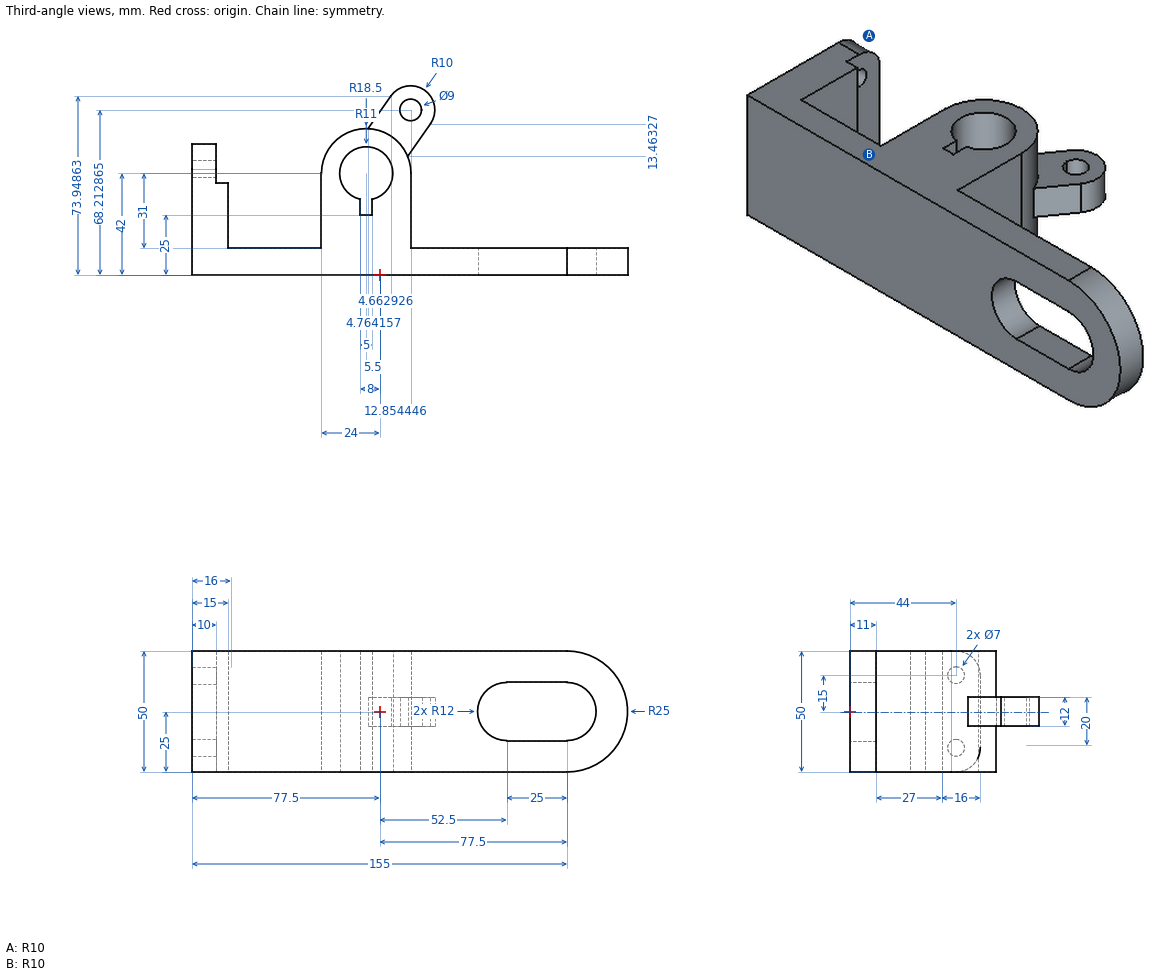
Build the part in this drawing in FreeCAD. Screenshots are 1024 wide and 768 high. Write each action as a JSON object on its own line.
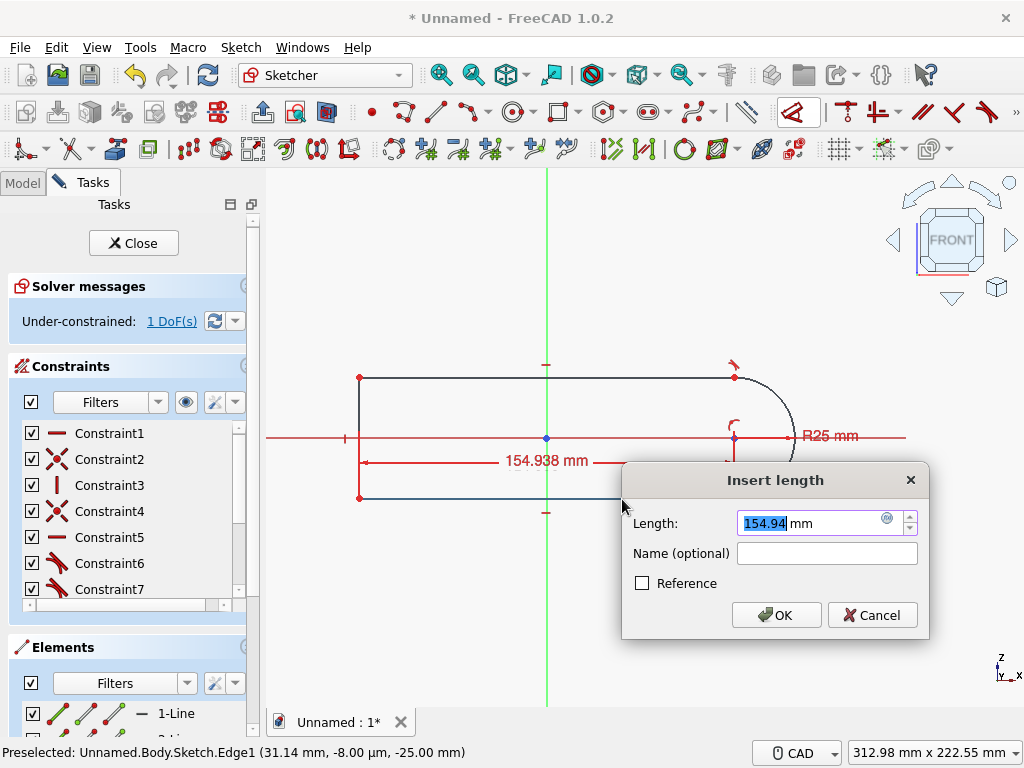
{"action": "type", "text": "155"}
{"action": "key", "text": "Return"}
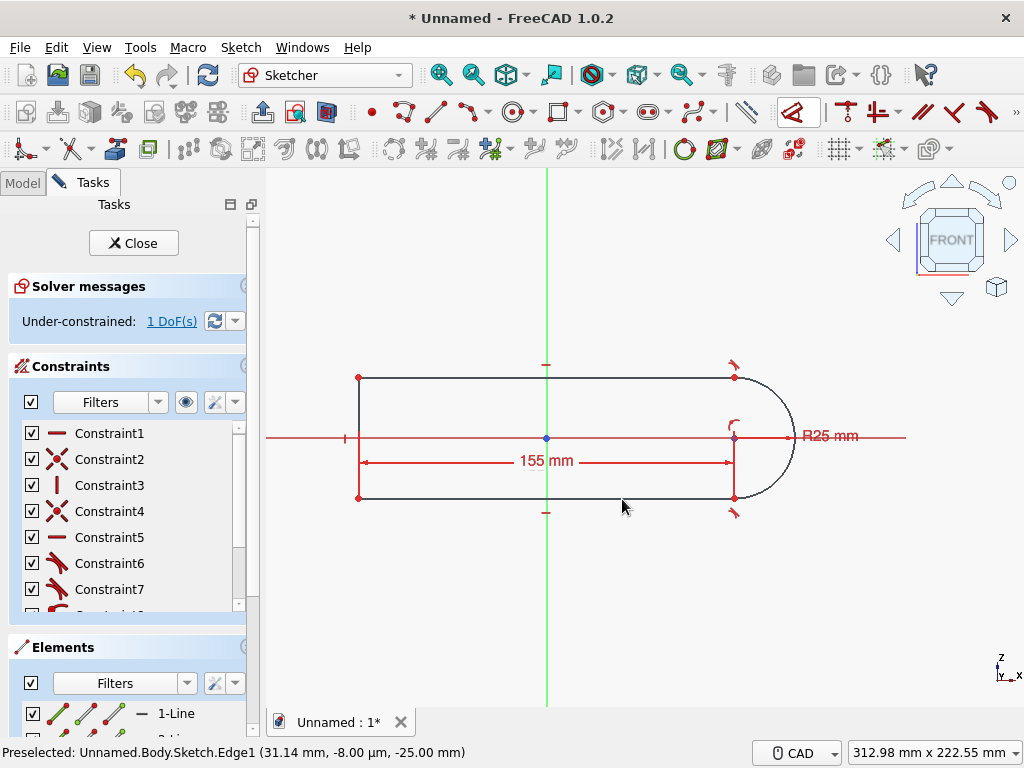
{"action": "left_click", "coordinate": [734, 499]}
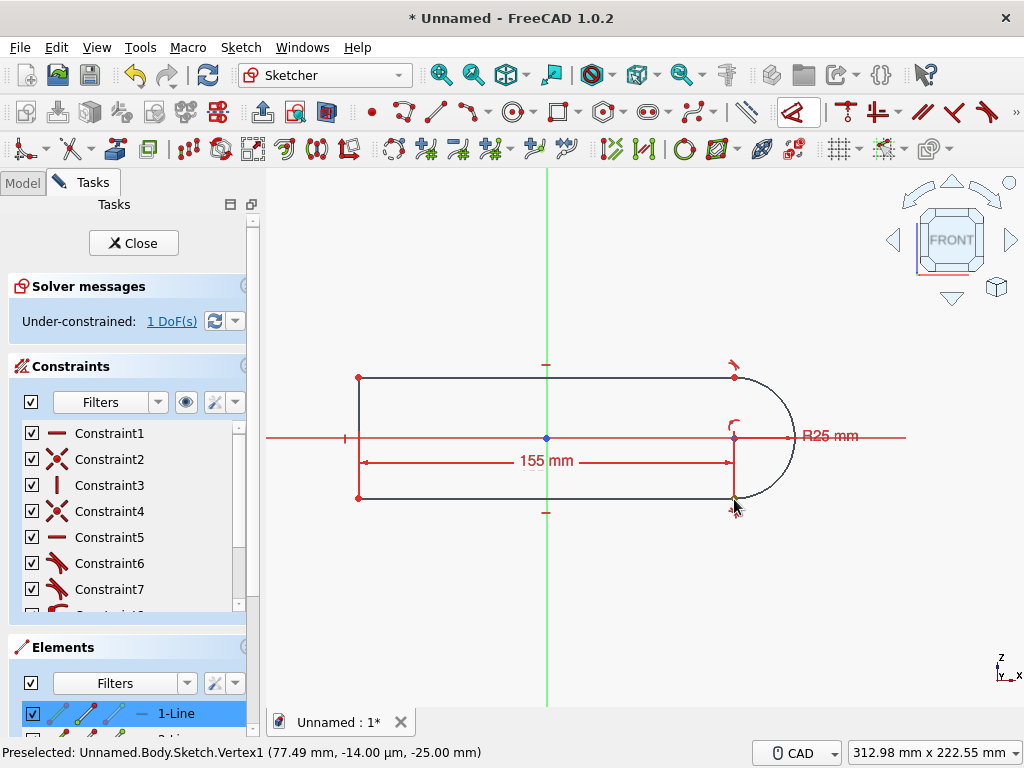
{"action": "left_click", "coordinate": [814, 112]}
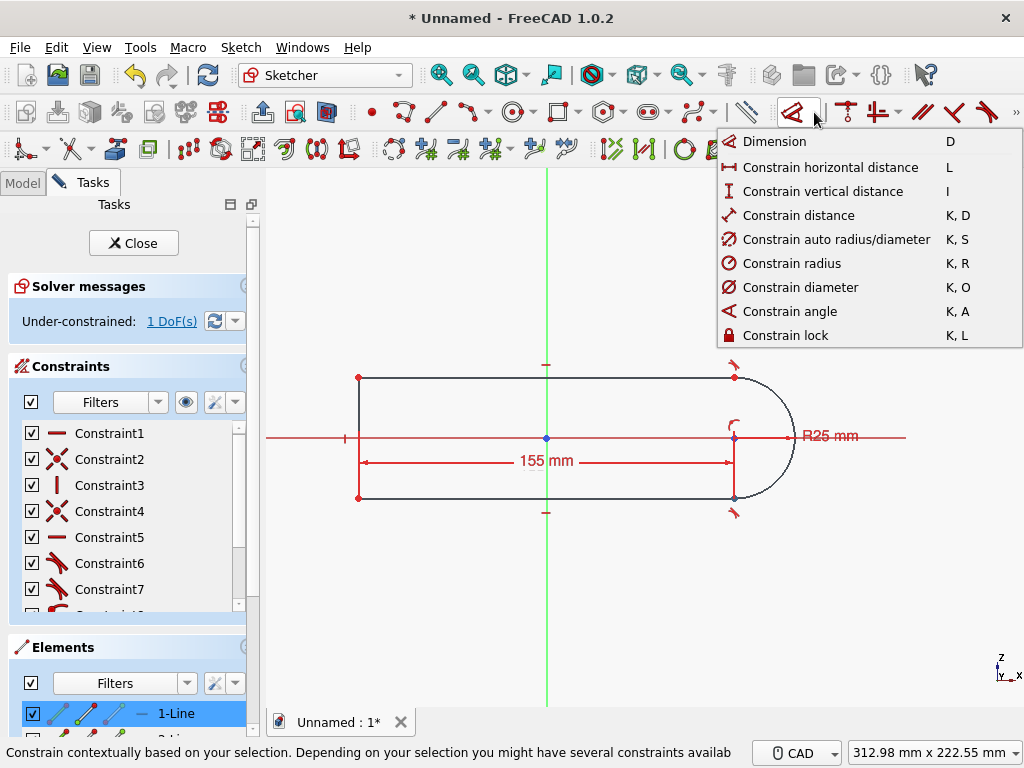
{"action": "left_click", "coordinate": [870, 167]}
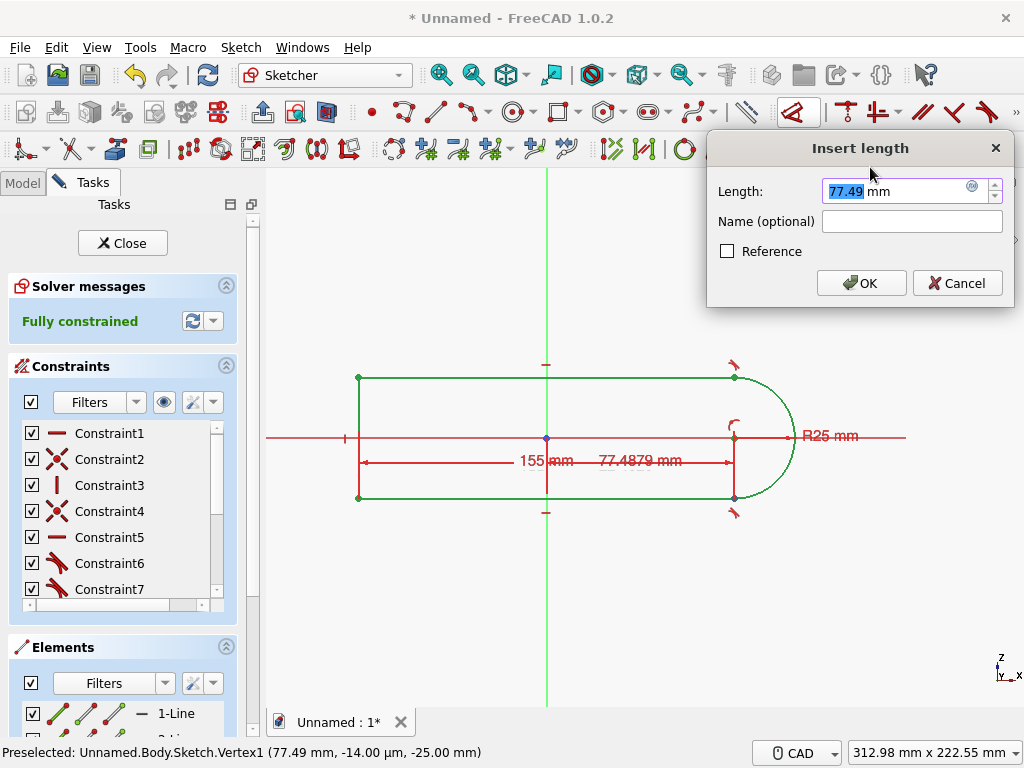
{"action": "type", "text": "77.5"}
{"action": "key", "text": "Return"}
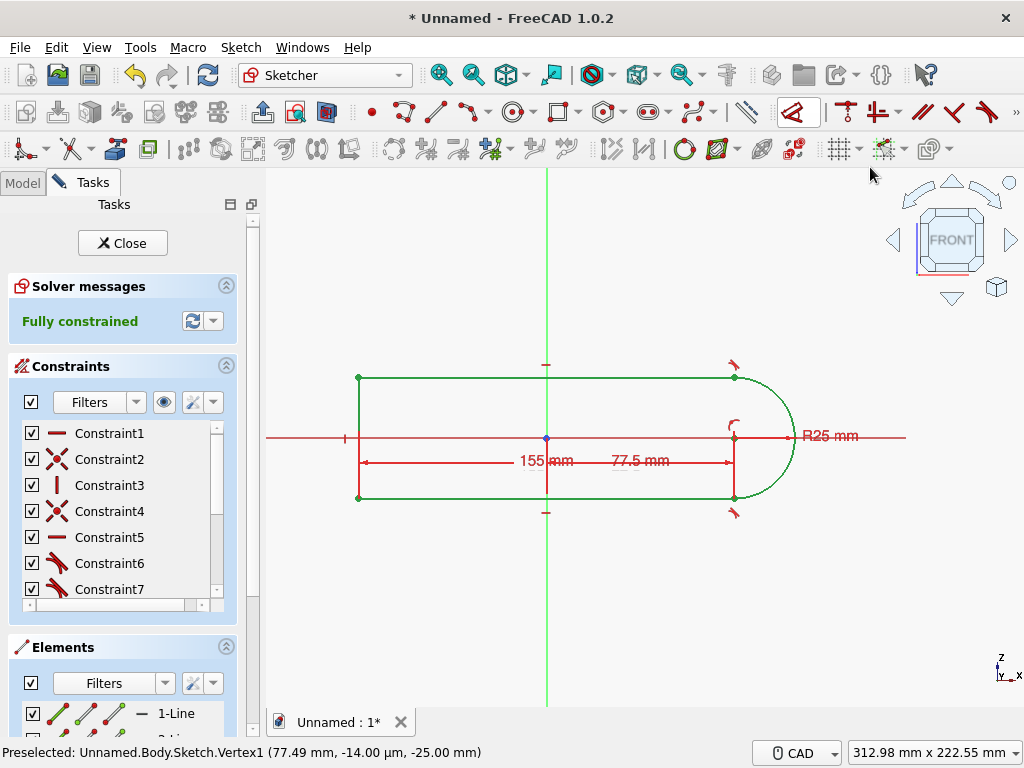
{"action": "left_click", "coordinate": [123, 243]}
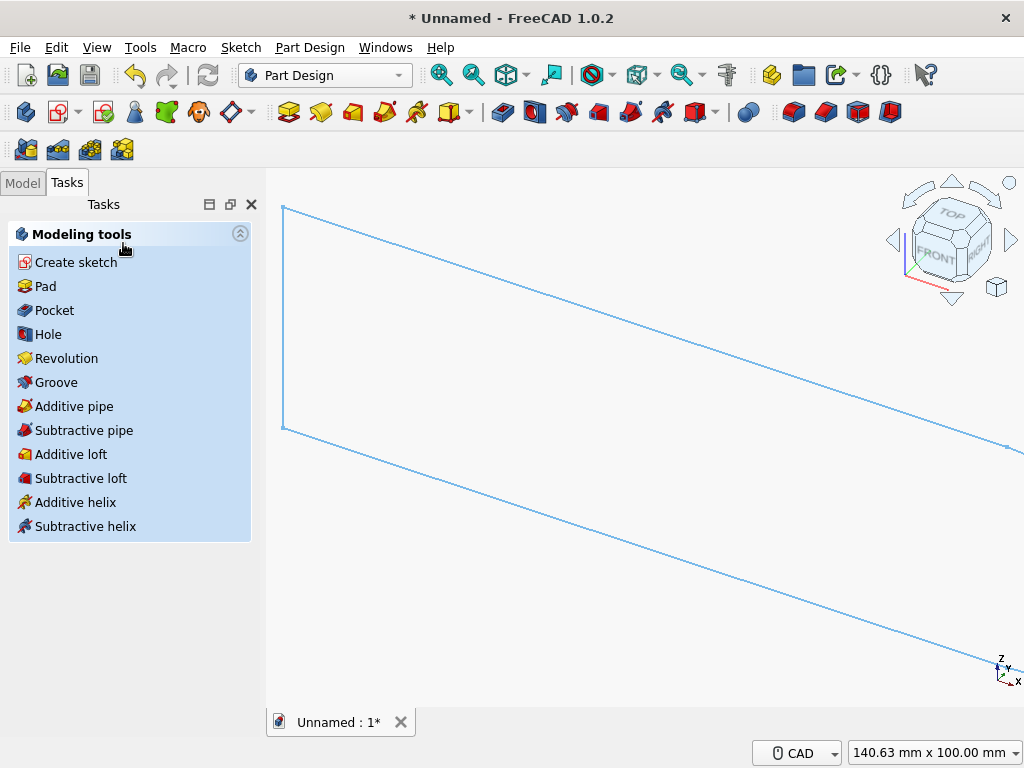
{"action": "left_click", "coordinate": [290, 112]}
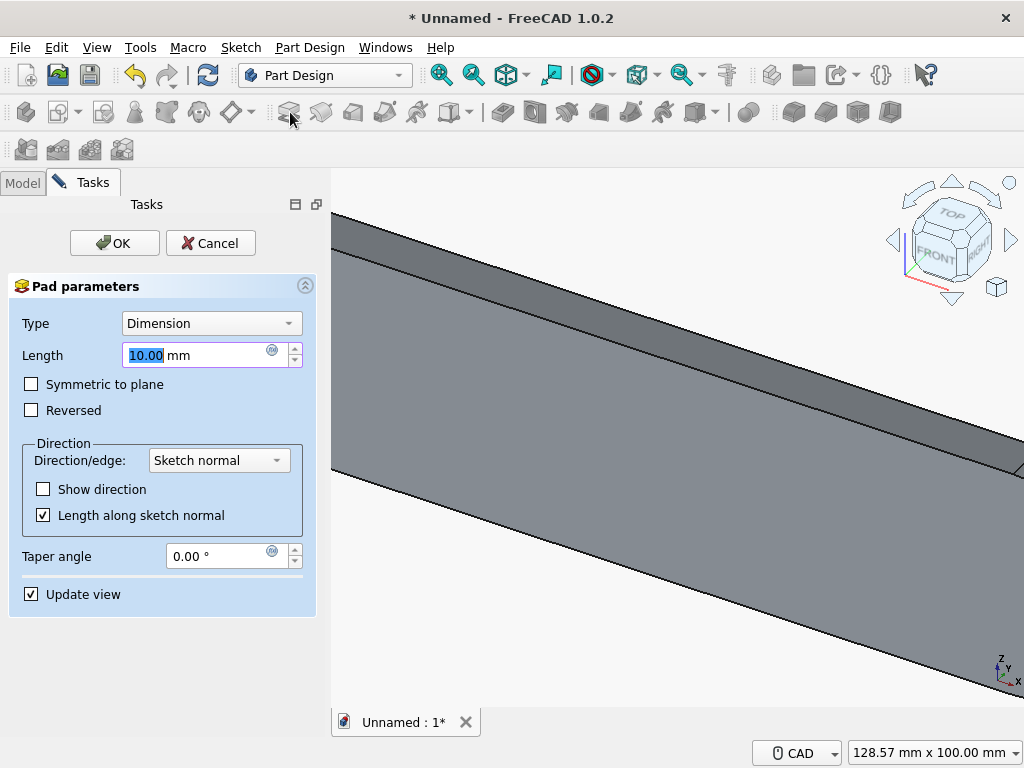
{"action": "type", "text": "11"}
{"action": "key", "text": "Tab"}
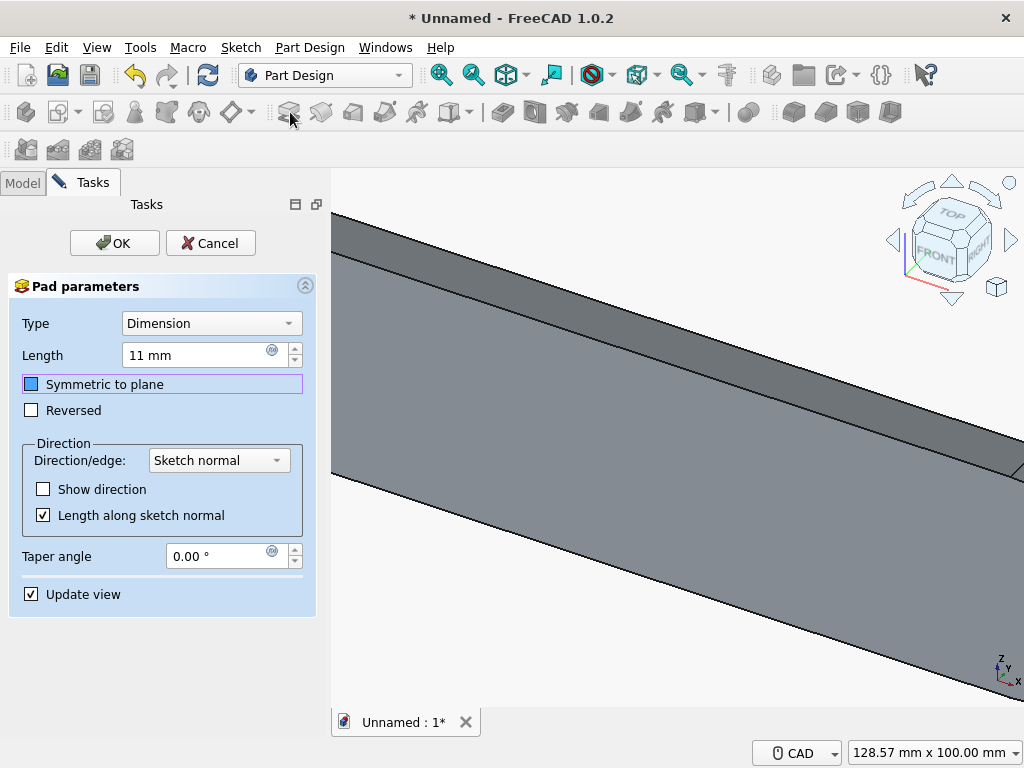
{"action": "left_click", "coordinate": [30, 410]}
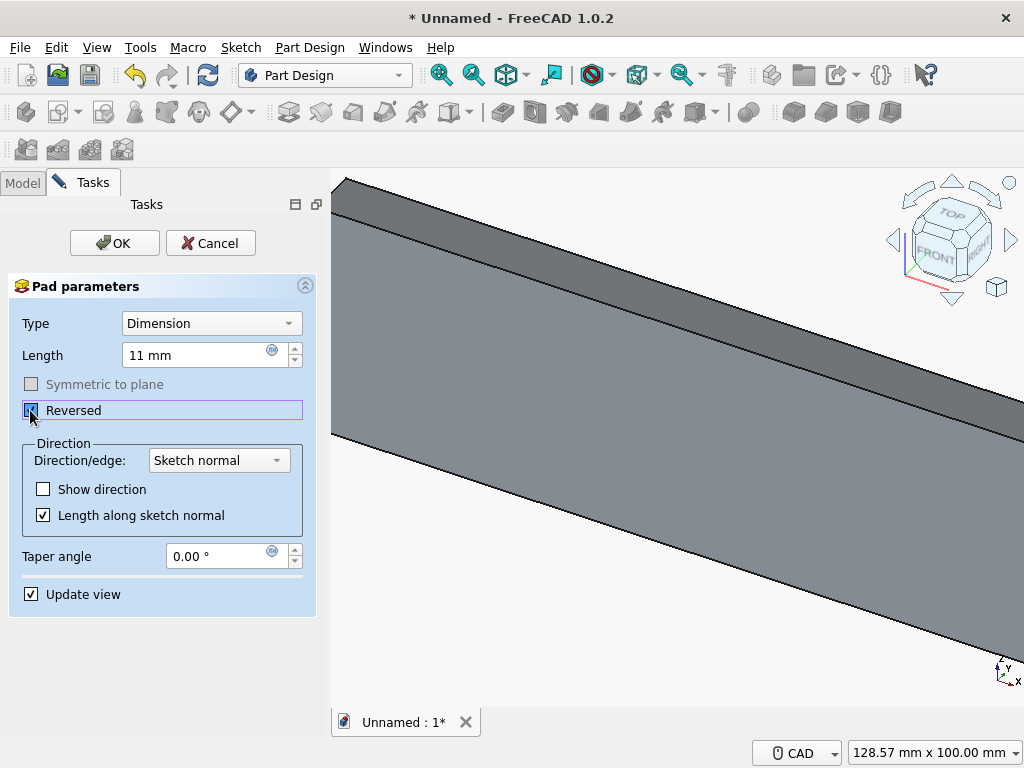
{"action": "left_click", "coordinate": [115, 243]}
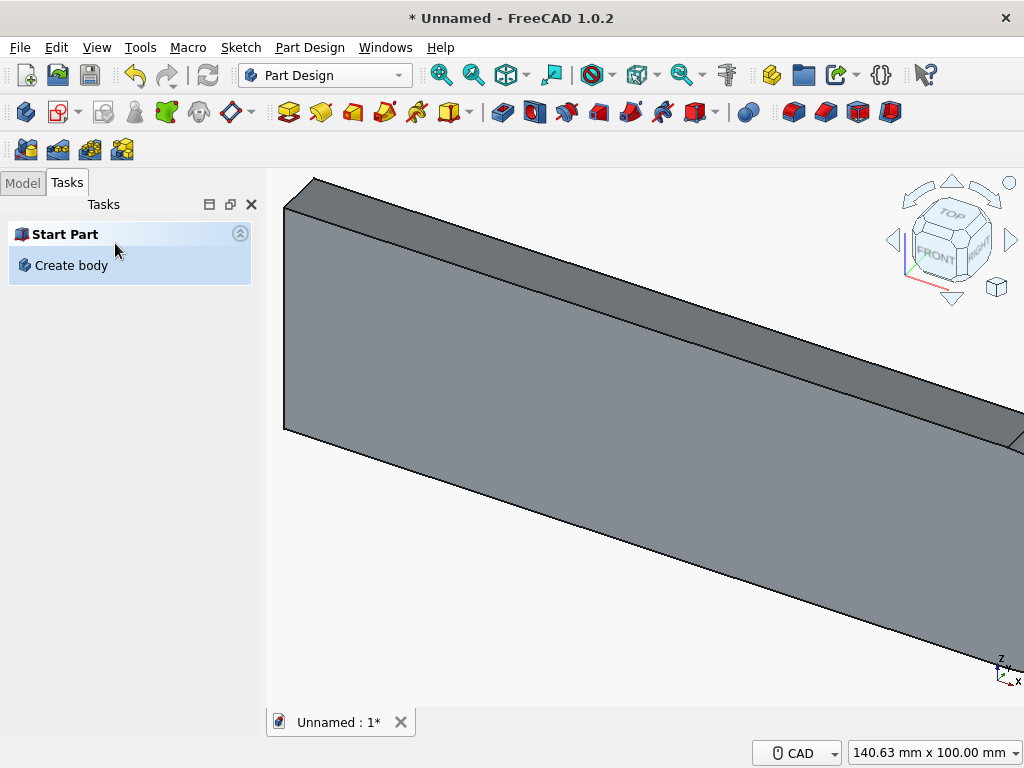
{"action": "left_click", "coordinate": [442, 76]}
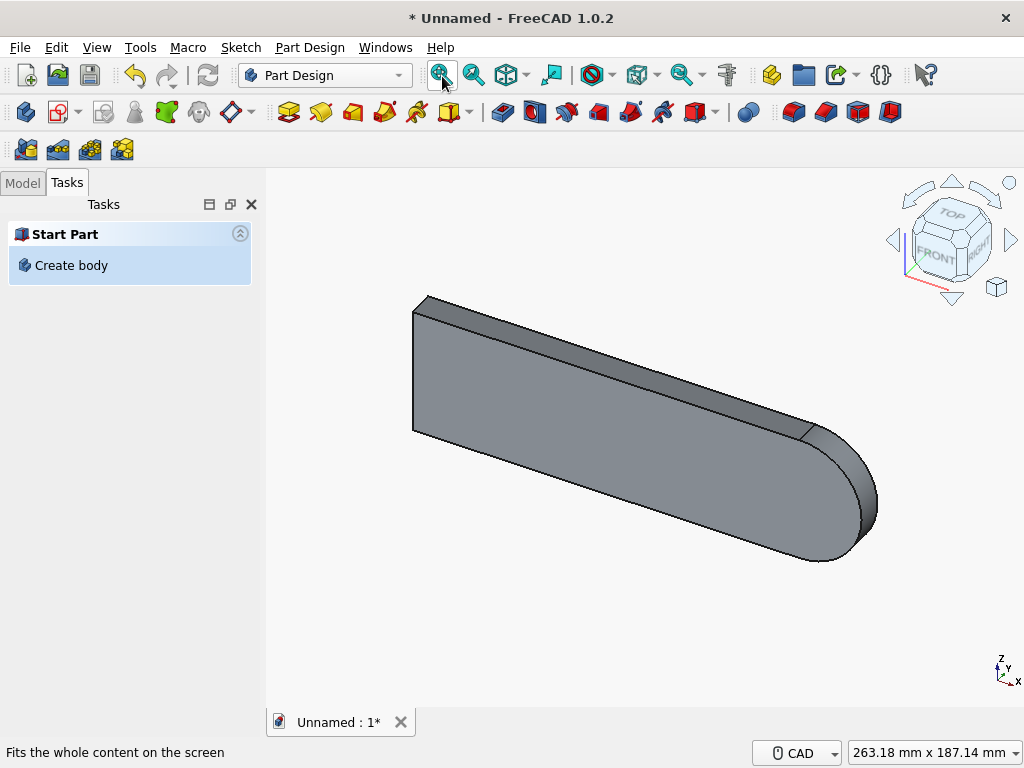
{"action": "key", "text": "4"}